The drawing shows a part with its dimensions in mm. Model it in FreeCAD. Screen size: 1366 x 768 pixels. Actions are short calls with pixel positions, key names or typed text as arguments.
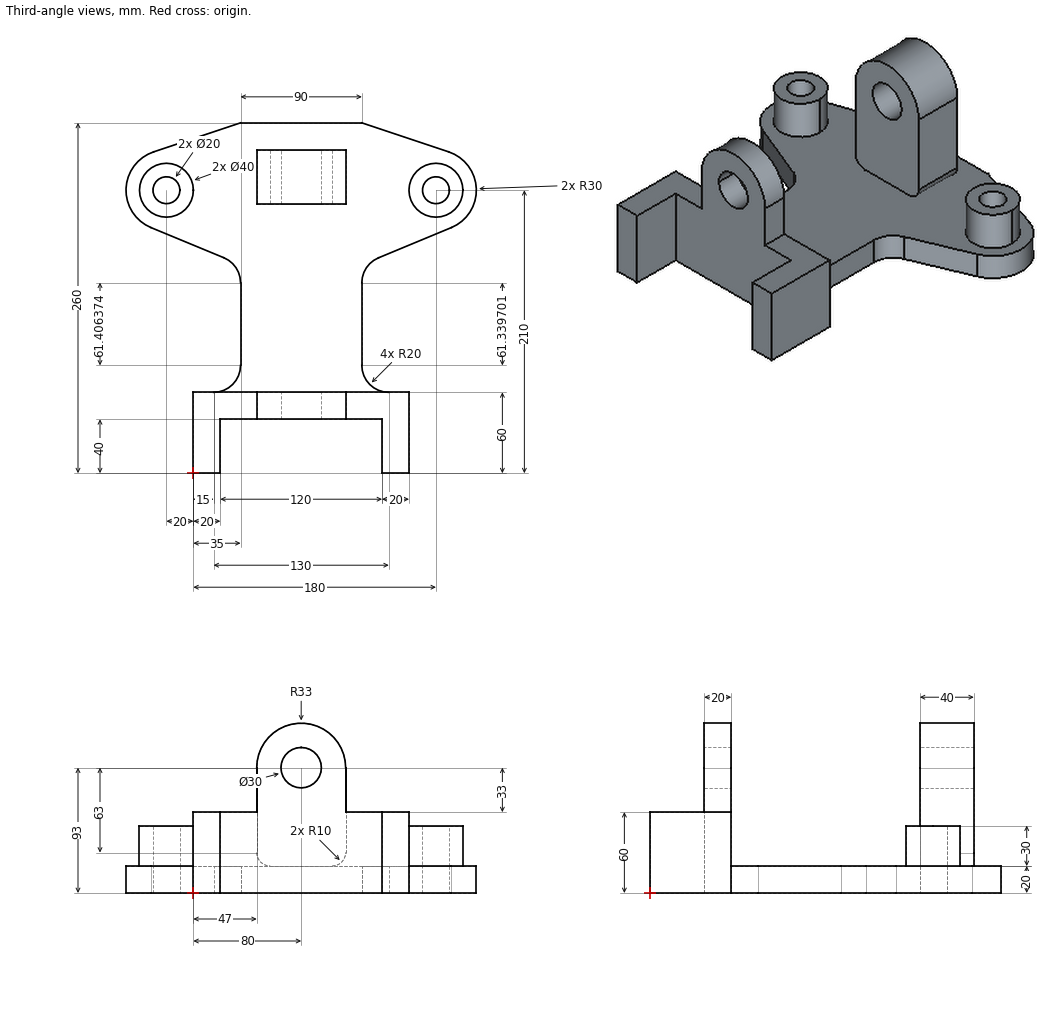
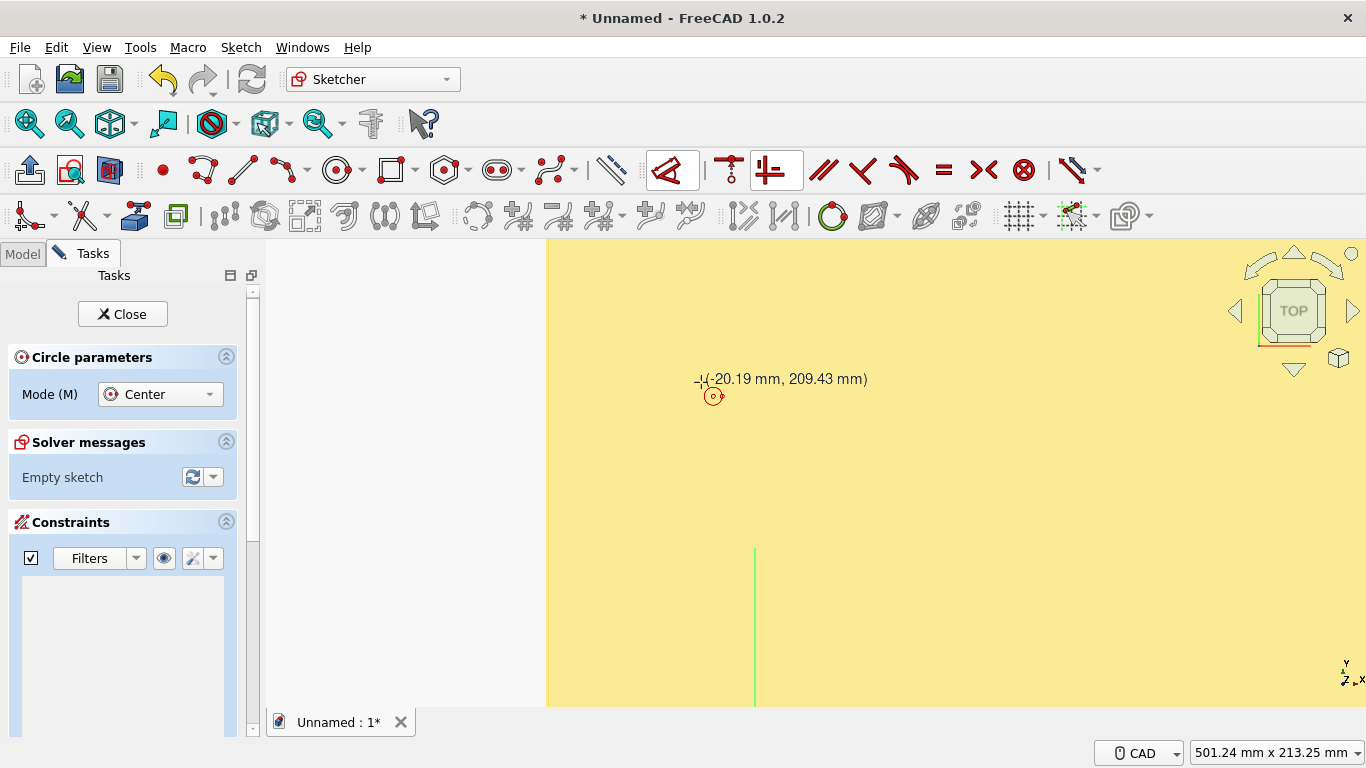
click(701, 382)
click(720, 363)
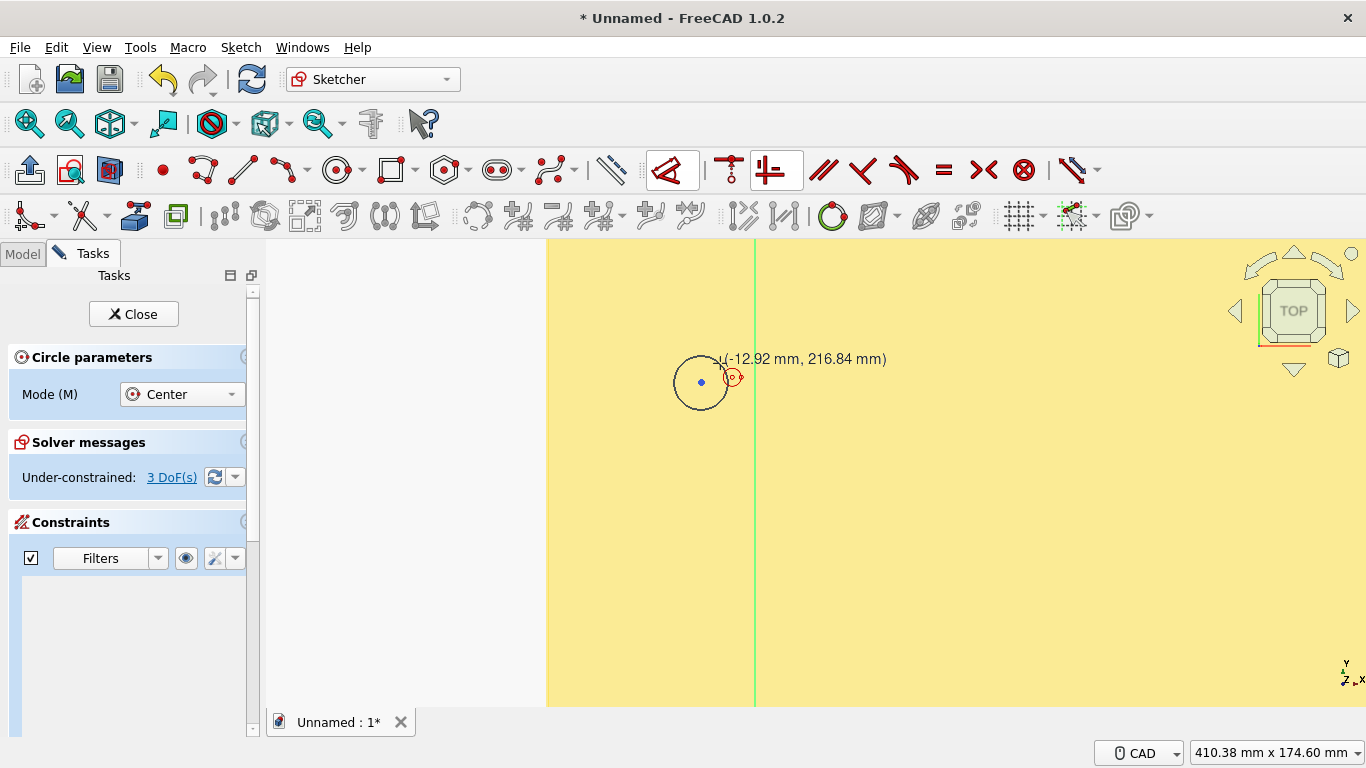
scroll(567, 328, down, 4)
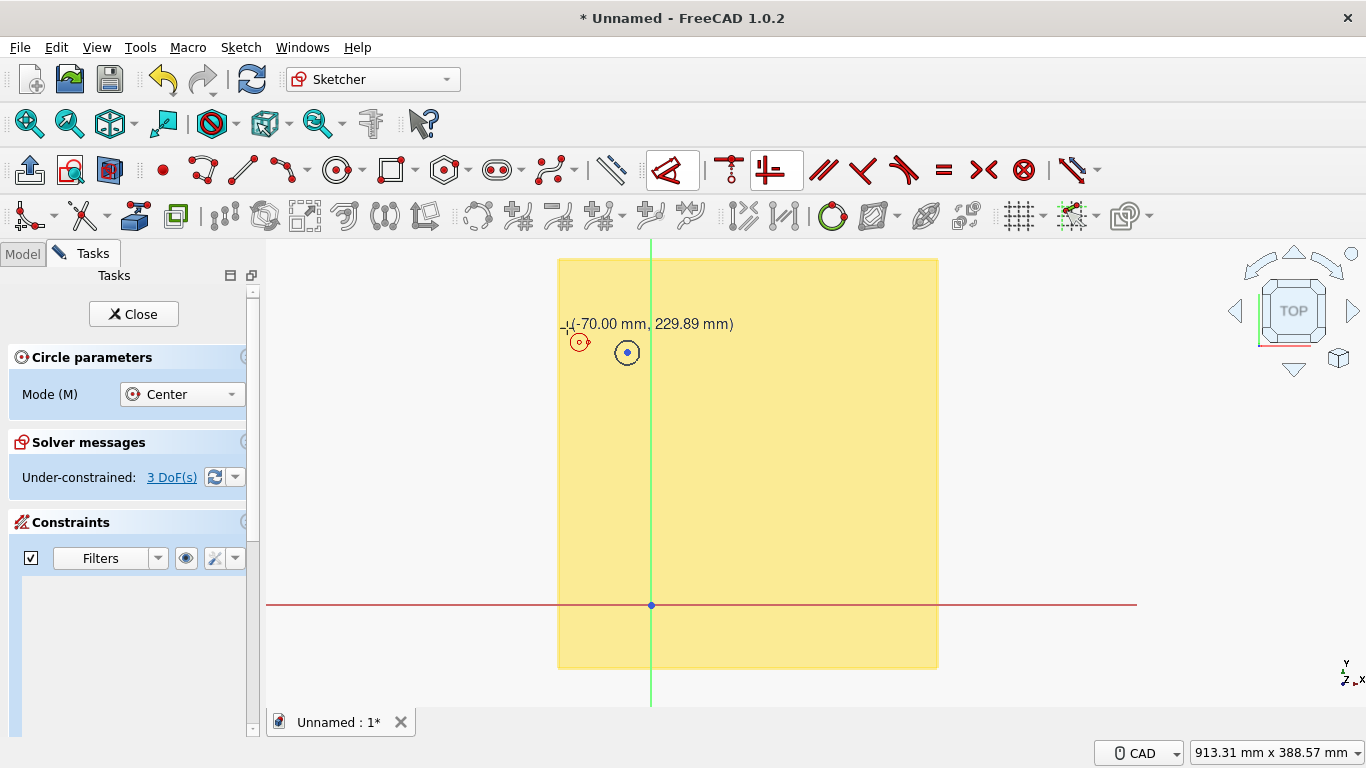
scroll(868, 353, up, 4)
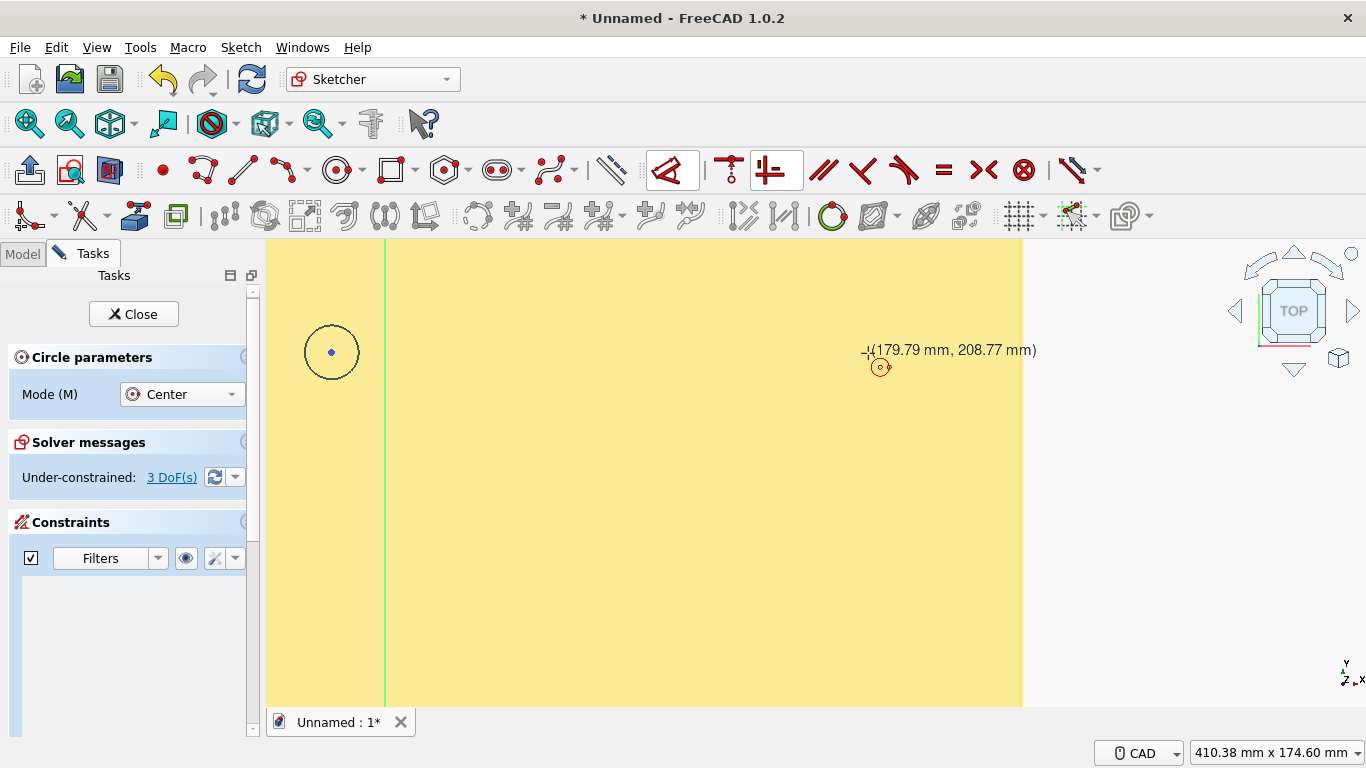
click(868, 352)
click(887, 333)
key(Escape)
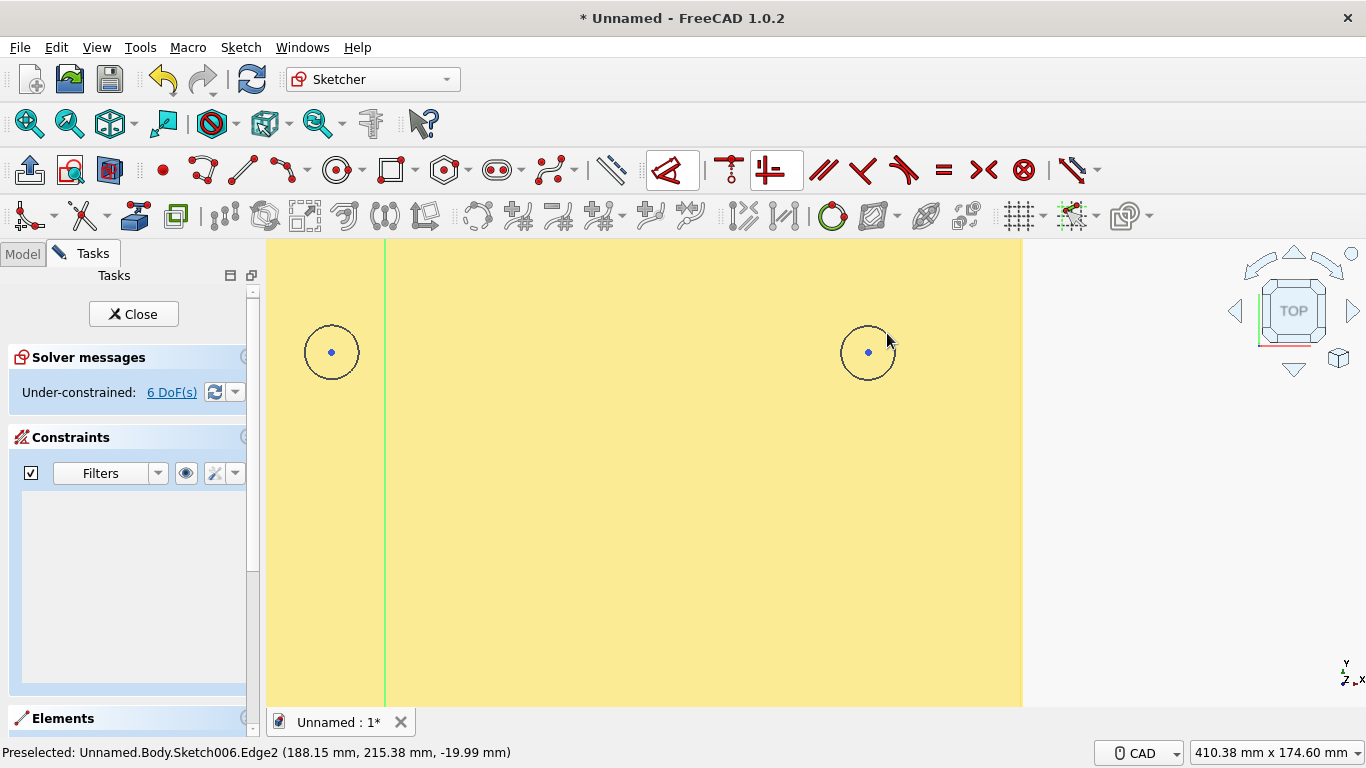
click(351, 333)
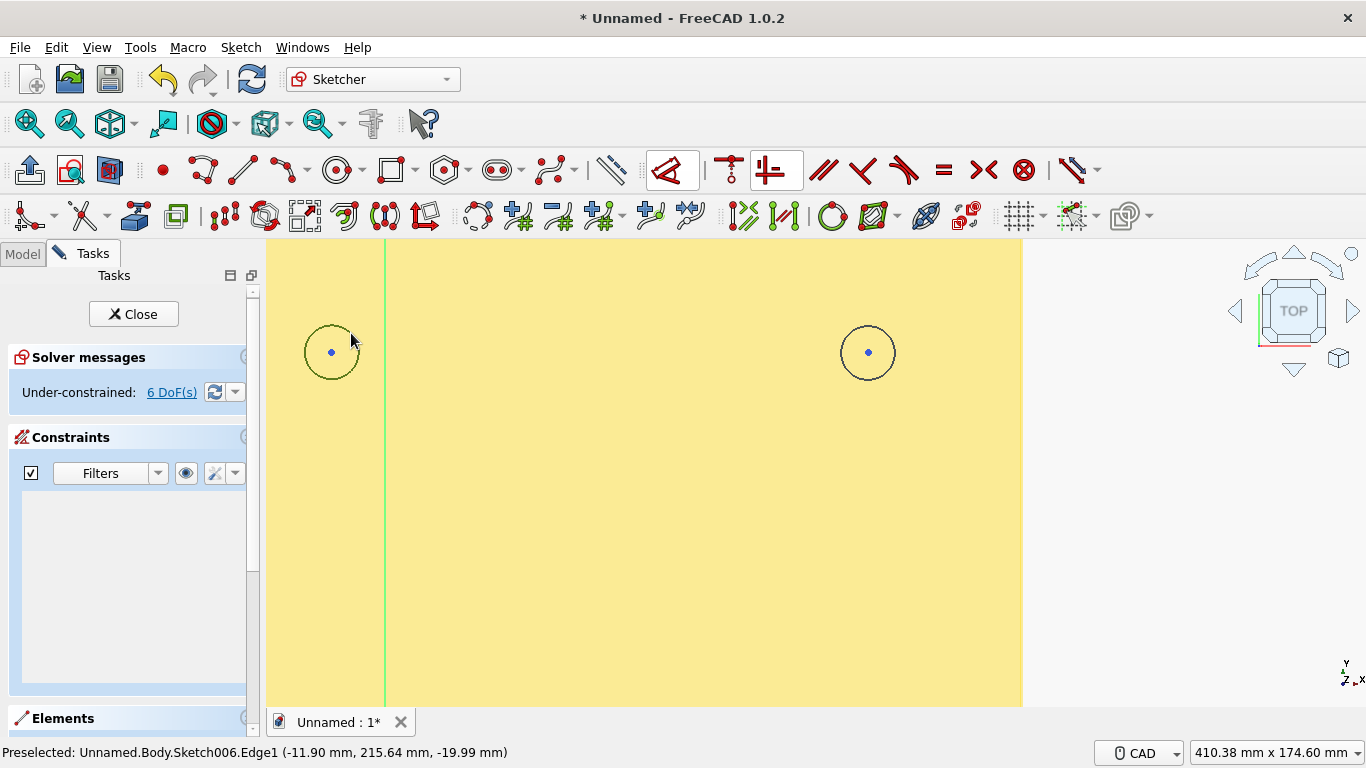
click(887, 334)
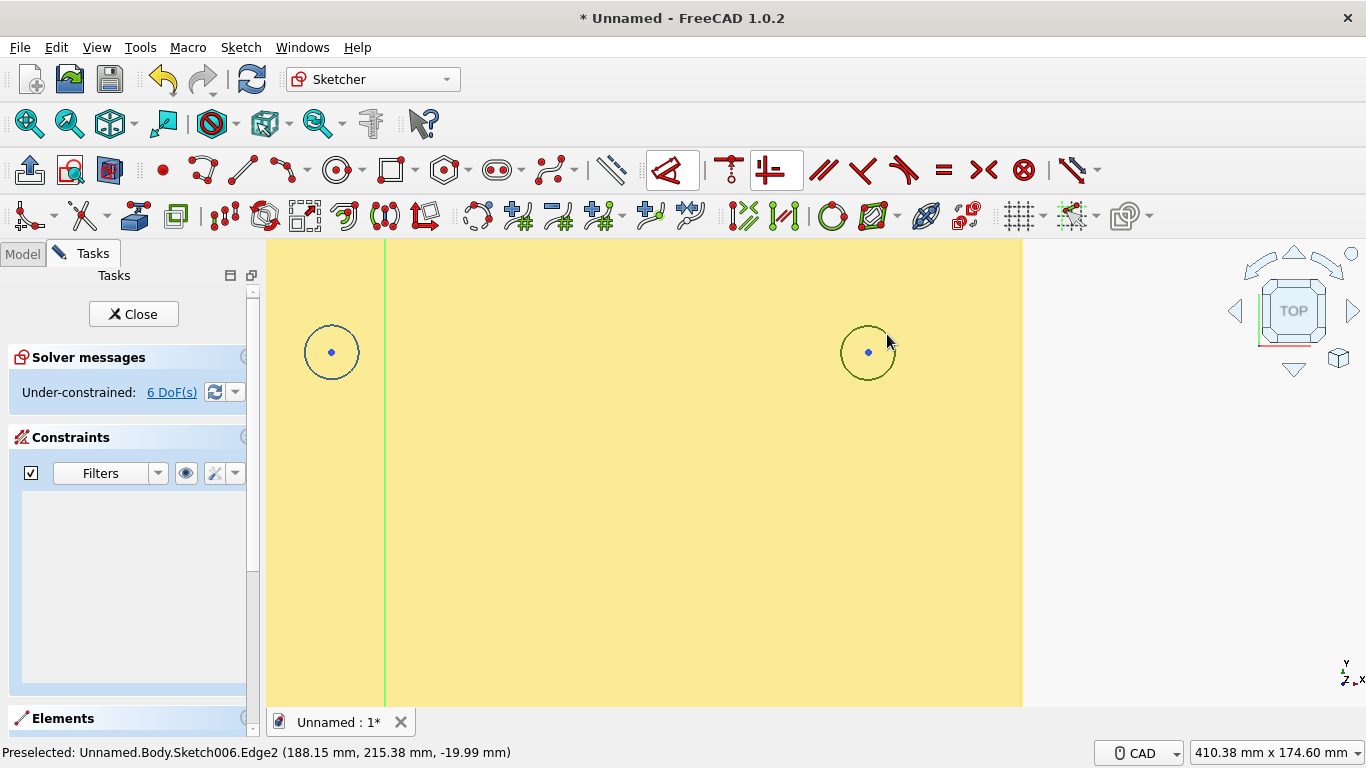
click(944, 170)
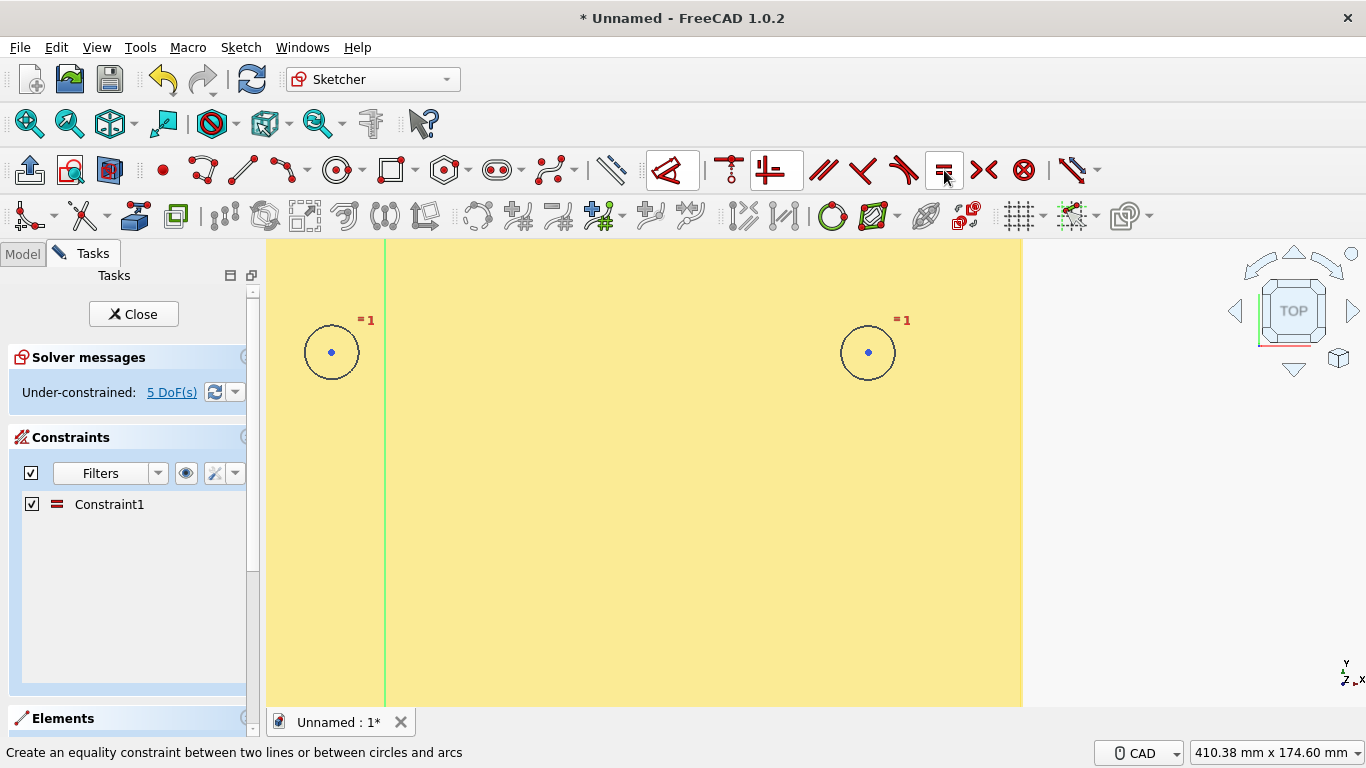
click(332, 352)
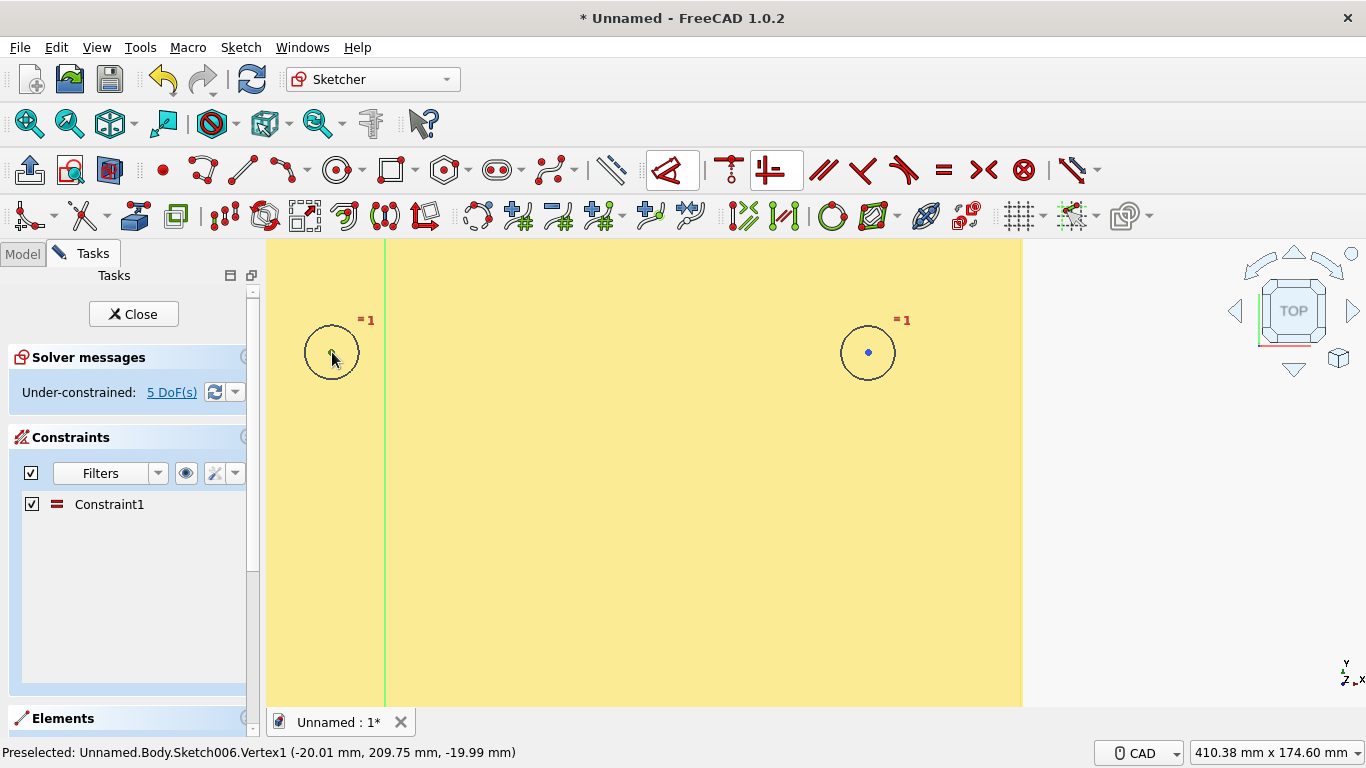
click(868, 353)